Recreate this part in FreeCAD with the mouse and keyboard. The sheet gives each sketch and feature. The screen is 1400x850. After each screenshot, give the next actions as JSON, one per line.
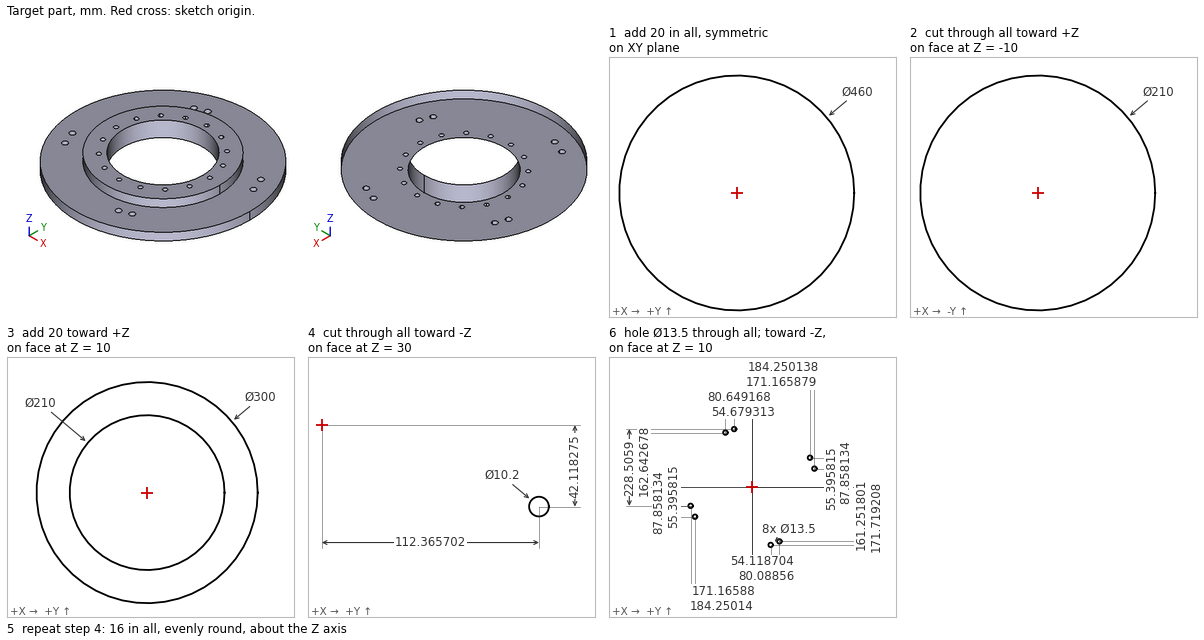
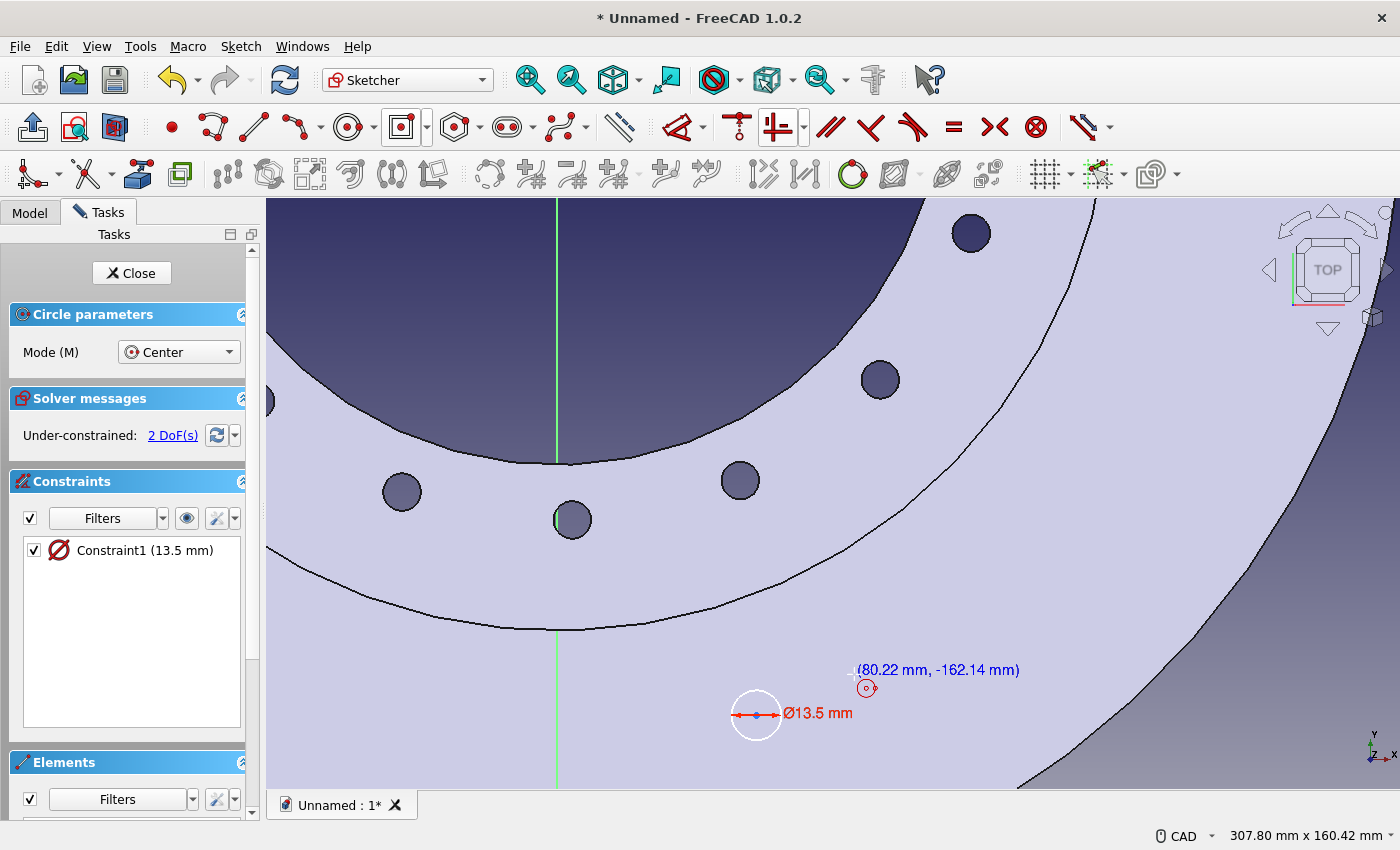
{"action": "scroll", "coordinate": [854, 674], "scroll_direction": "down", "scroll_amount": 6}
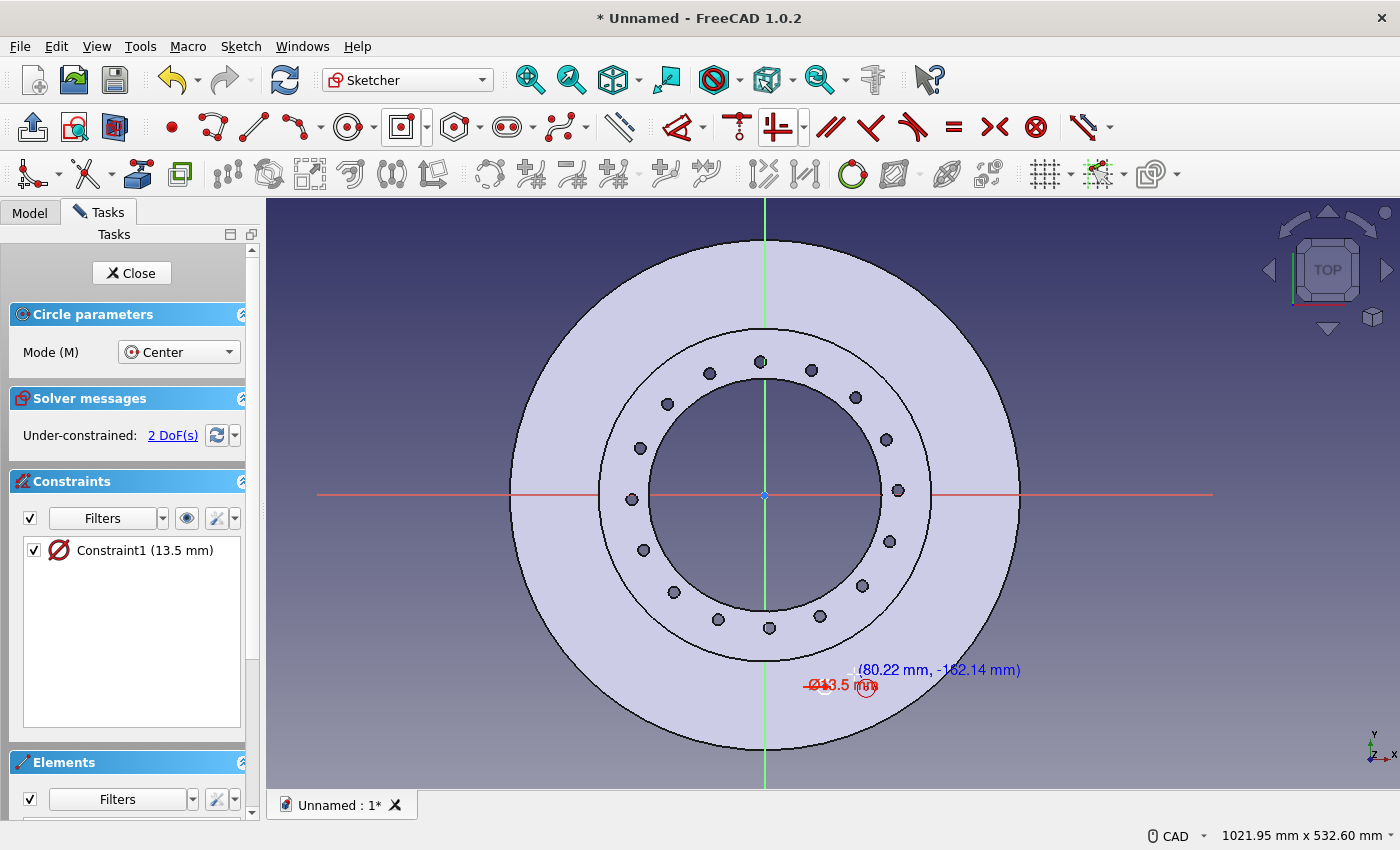
{"action": "left_click", "coordinate": [854, 674]}
{"action": "mouse_move", "coordinate": [859, 669]}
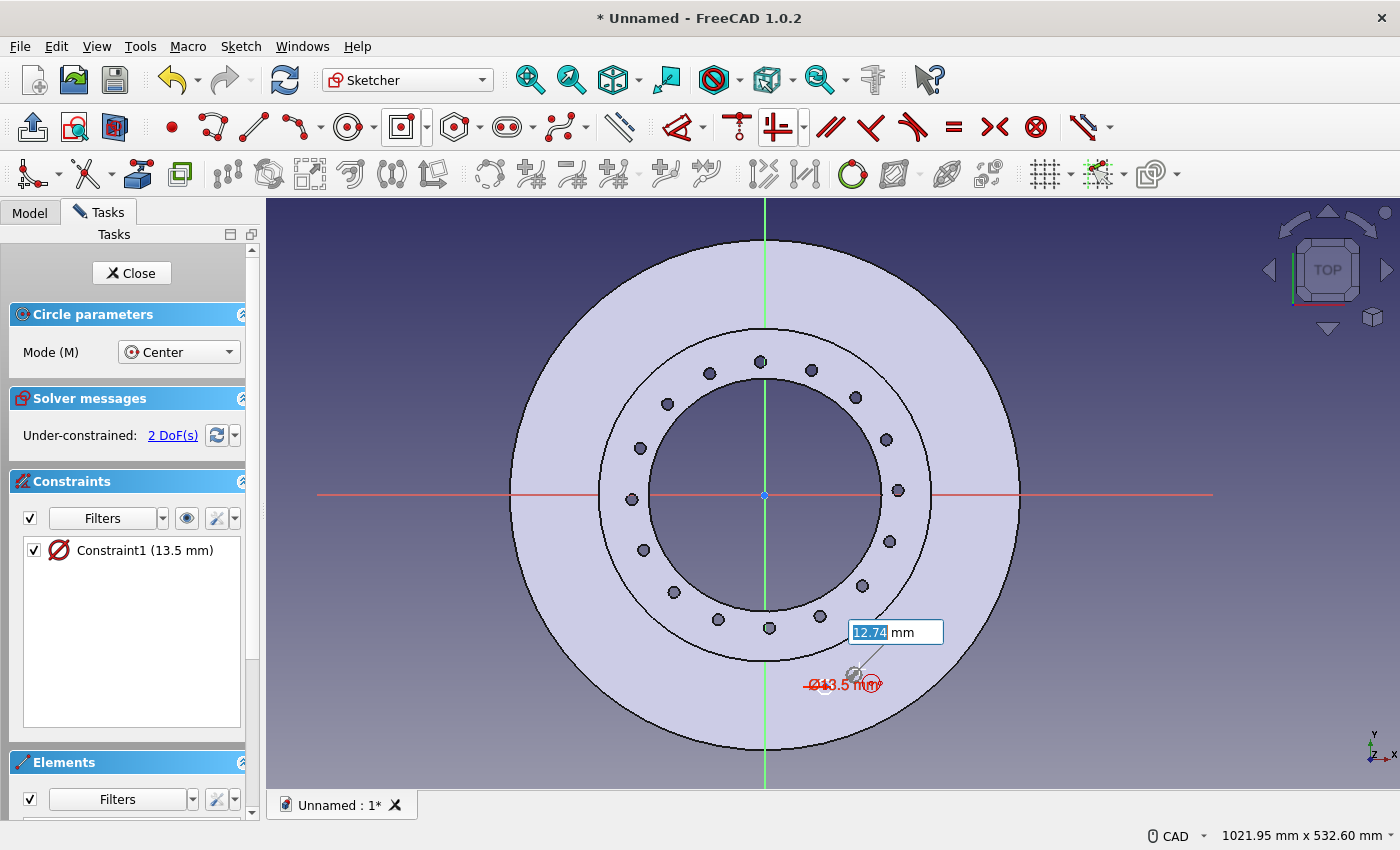
{"action": "type", "text": "13.5"}
{"action": "key", "text": "Return"}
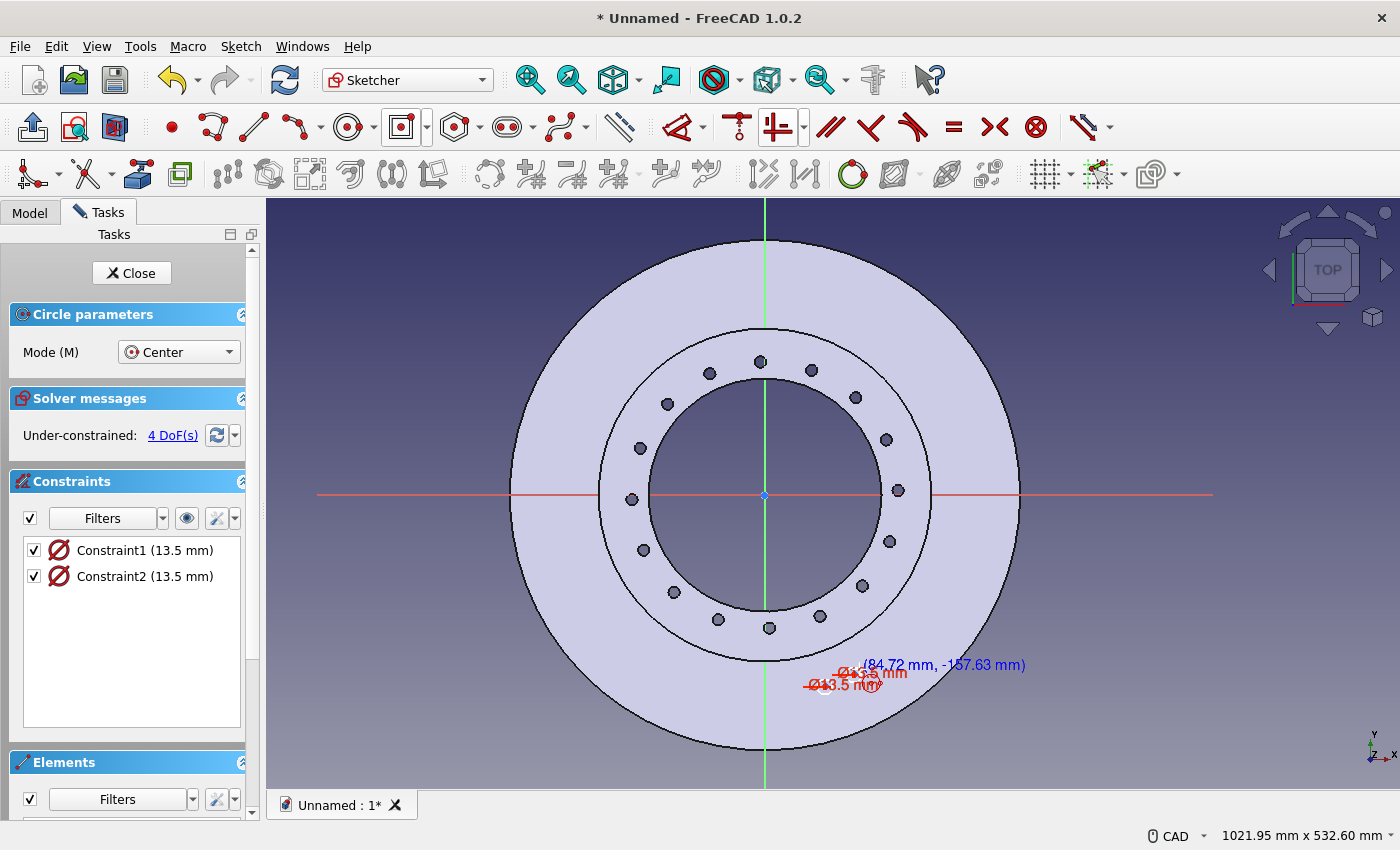
{"action": "scroll", "coordinate": [955, 398], "scroll_direction": "up", "scroll_amount": 6}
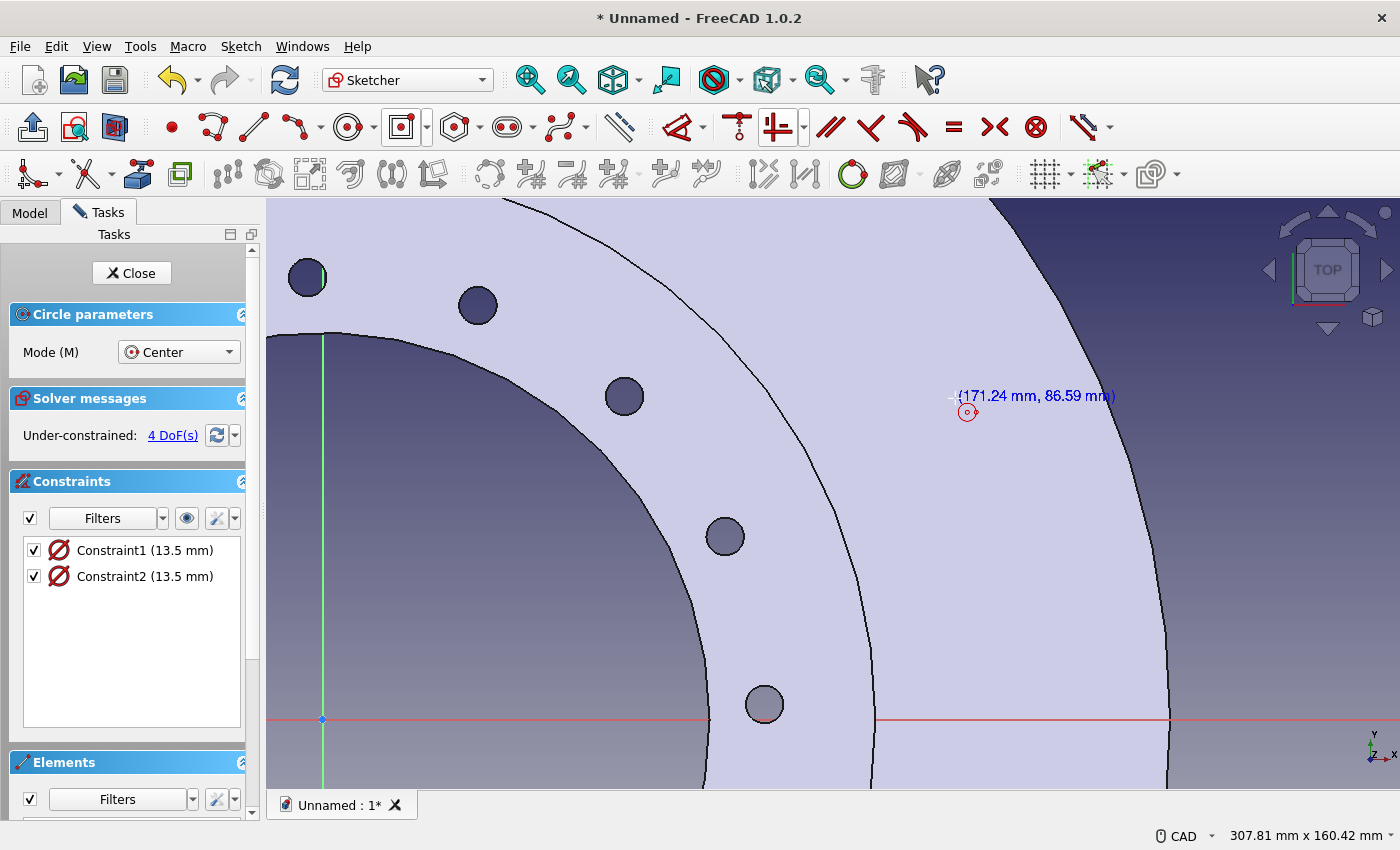
{"action": "scroll", "coordinate": [955, 397], "scroll_direction": "down", "scroll_amount": 6}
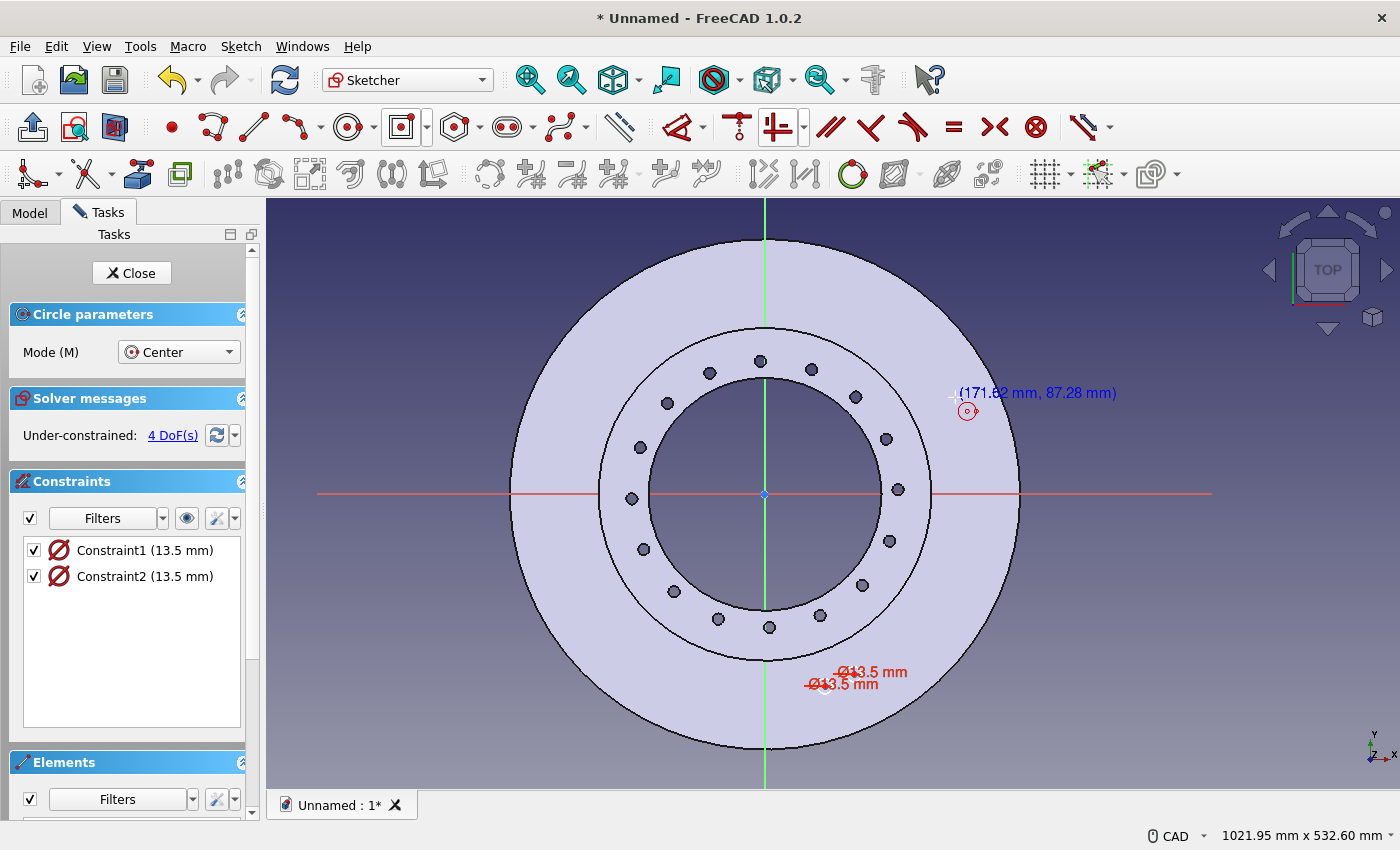
{"action": "left_click", "coordinate": [955, 397]}
{"action": "mouse_move", "coordinate": [960, 392]}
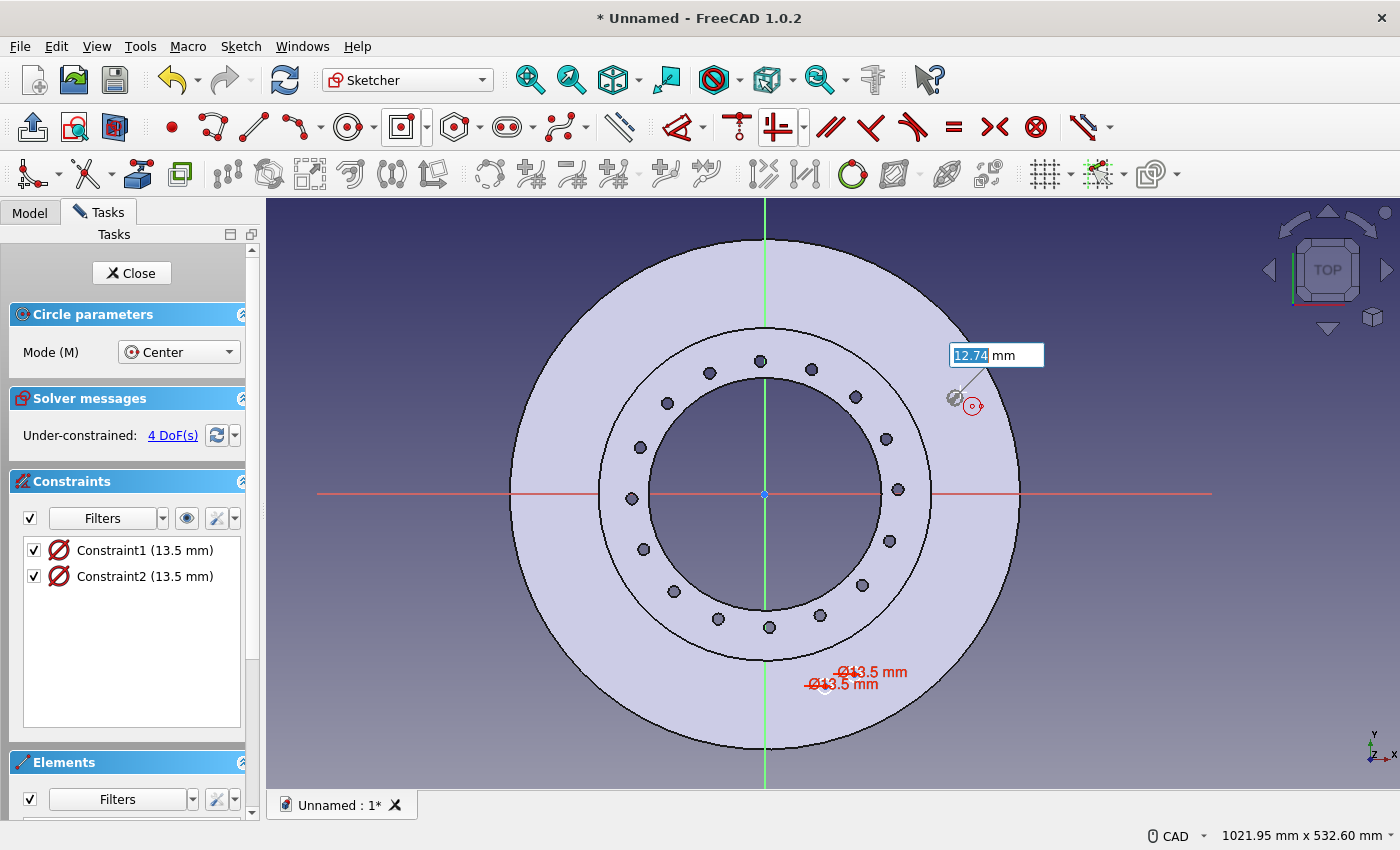
{"action": "type", "text": "13.5"}
{"action": "key", "text": "Return"}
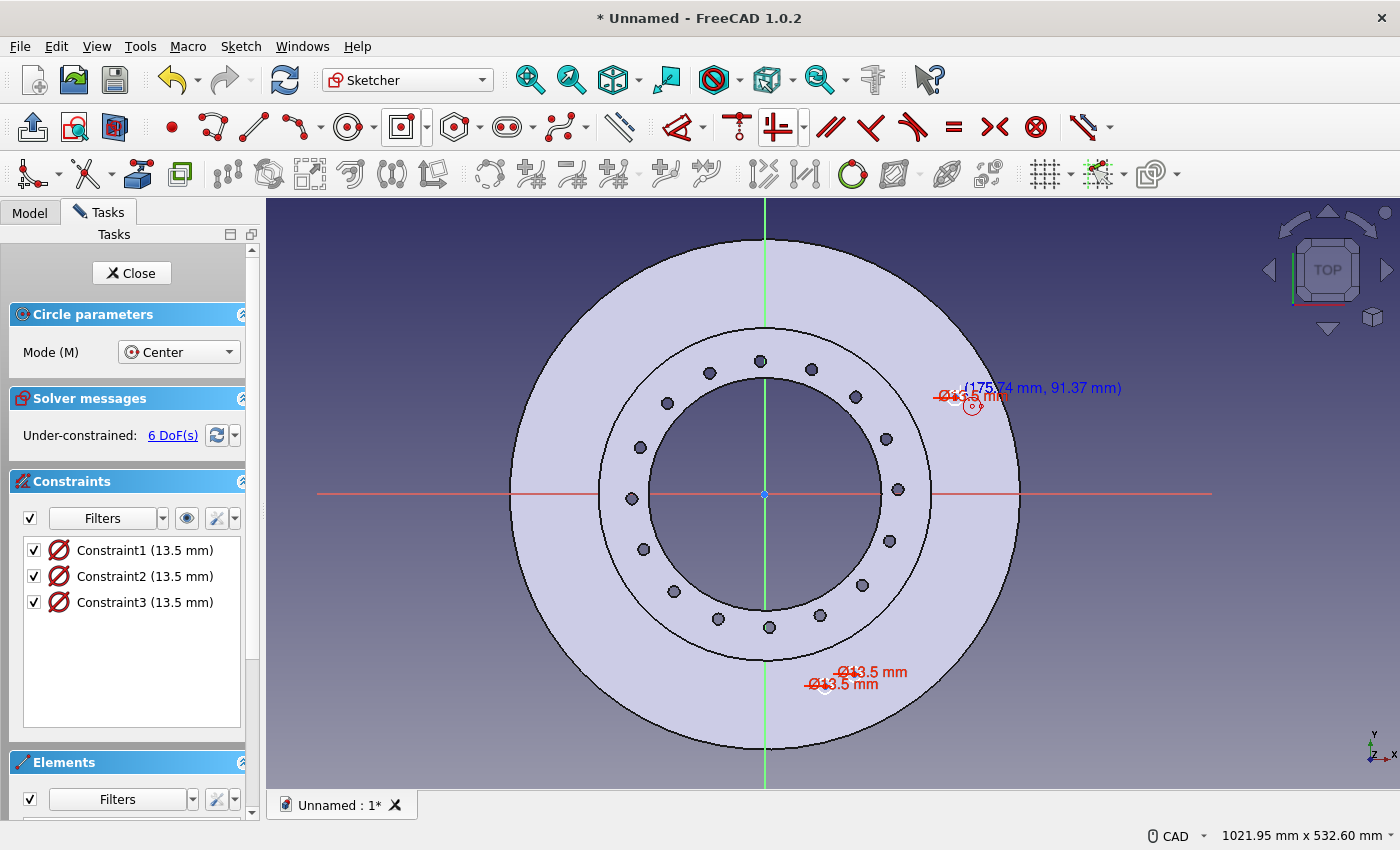
{"action": "scroll", "coordinate": [969, 433], "scroll_direction": "up", "scroll_amount": 6}